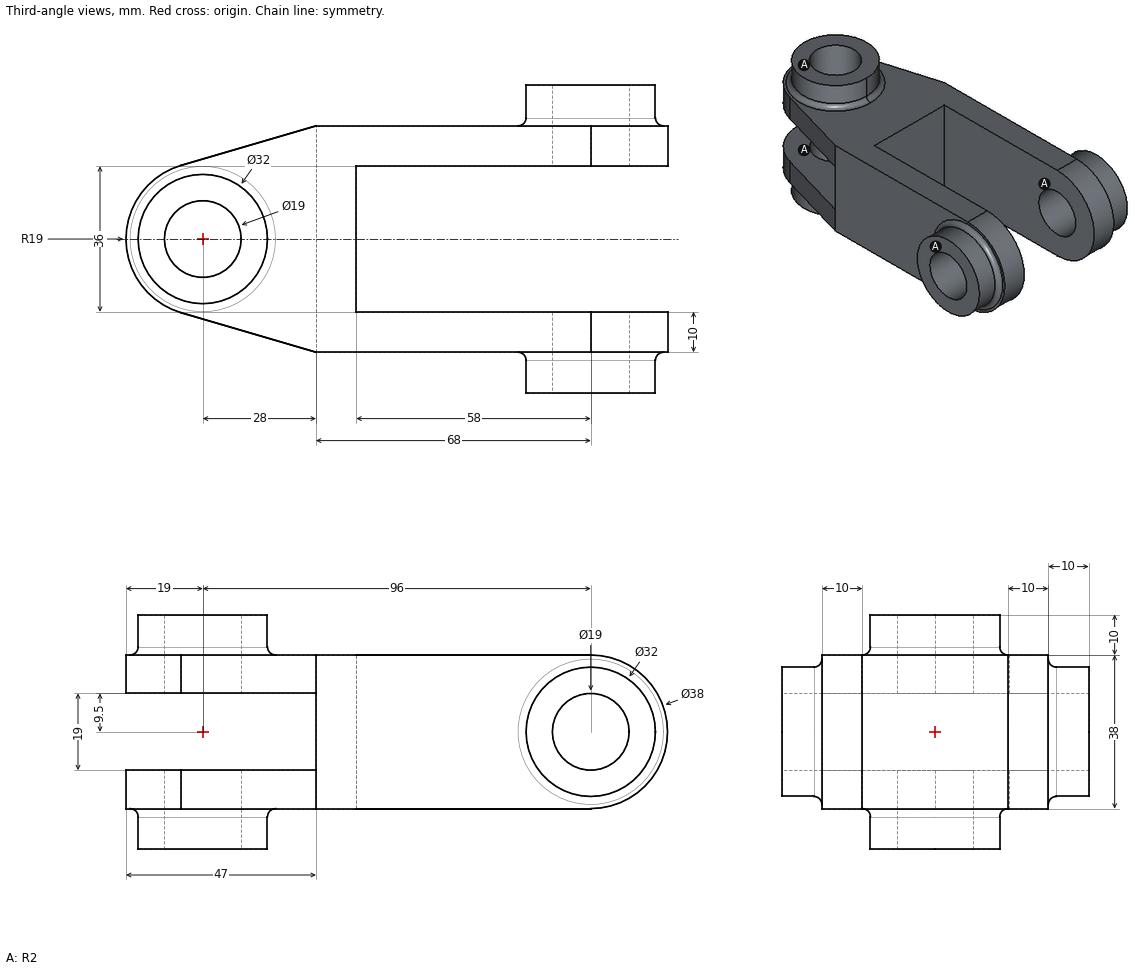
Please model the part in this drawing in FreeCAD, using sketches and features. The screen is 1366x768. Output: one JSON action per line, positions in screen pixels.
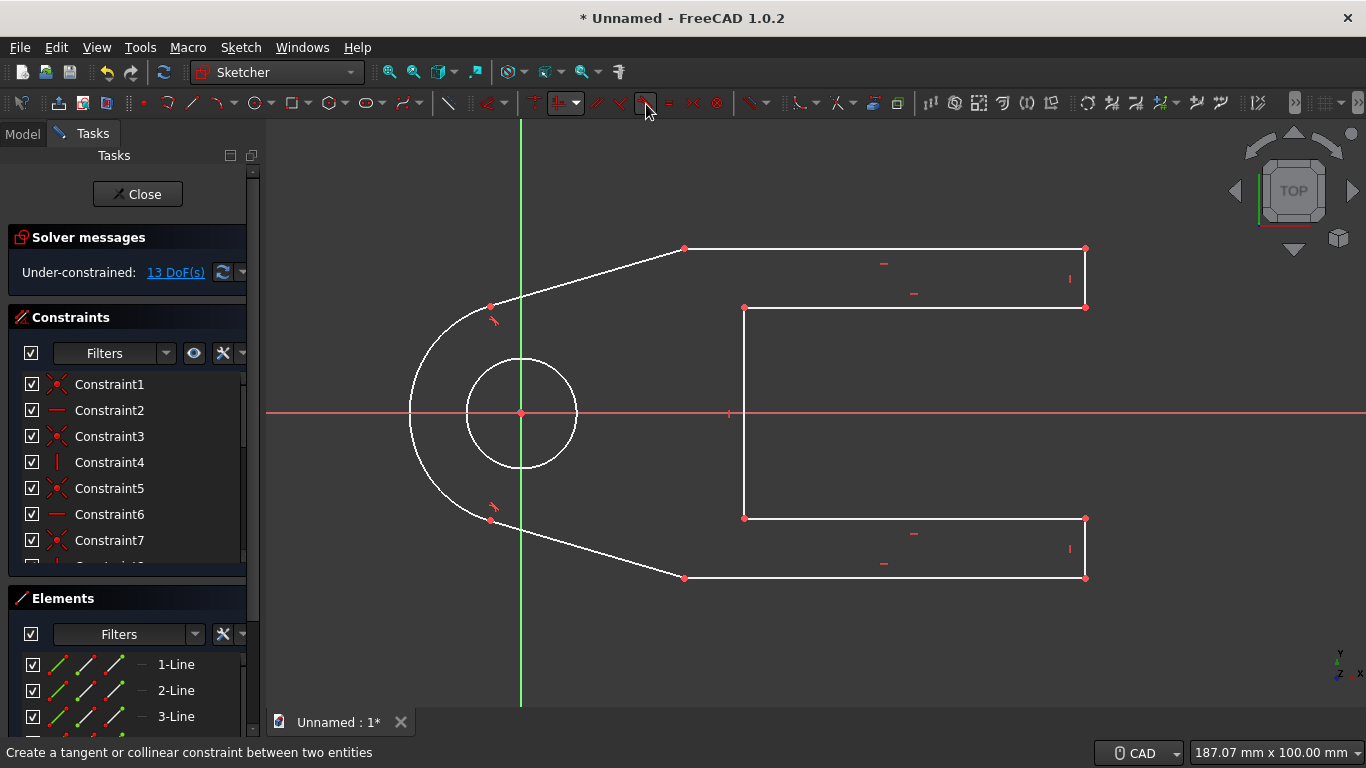
{"action": "left_click_drag", "start_coordinate": [511, 403], "coordinate": [532, 423]}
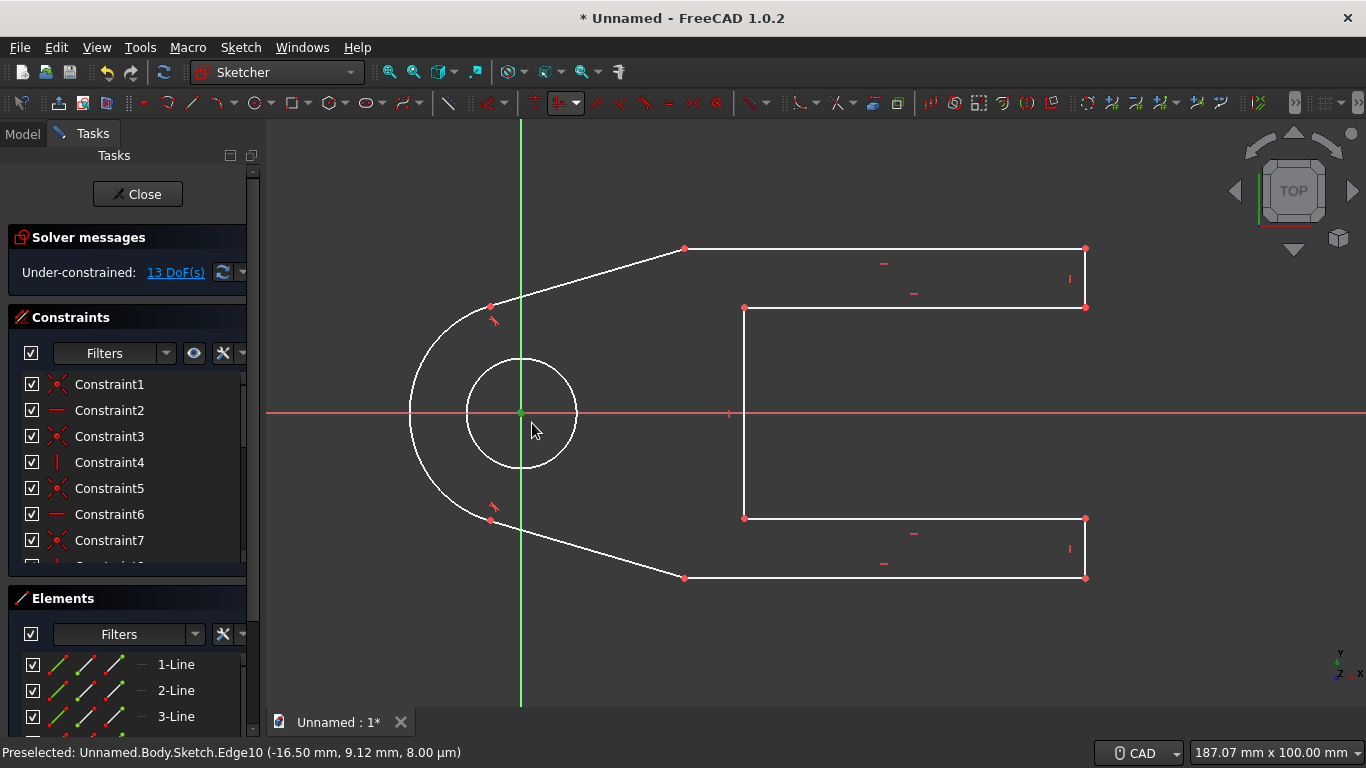
{"action": "key", "text": "c"}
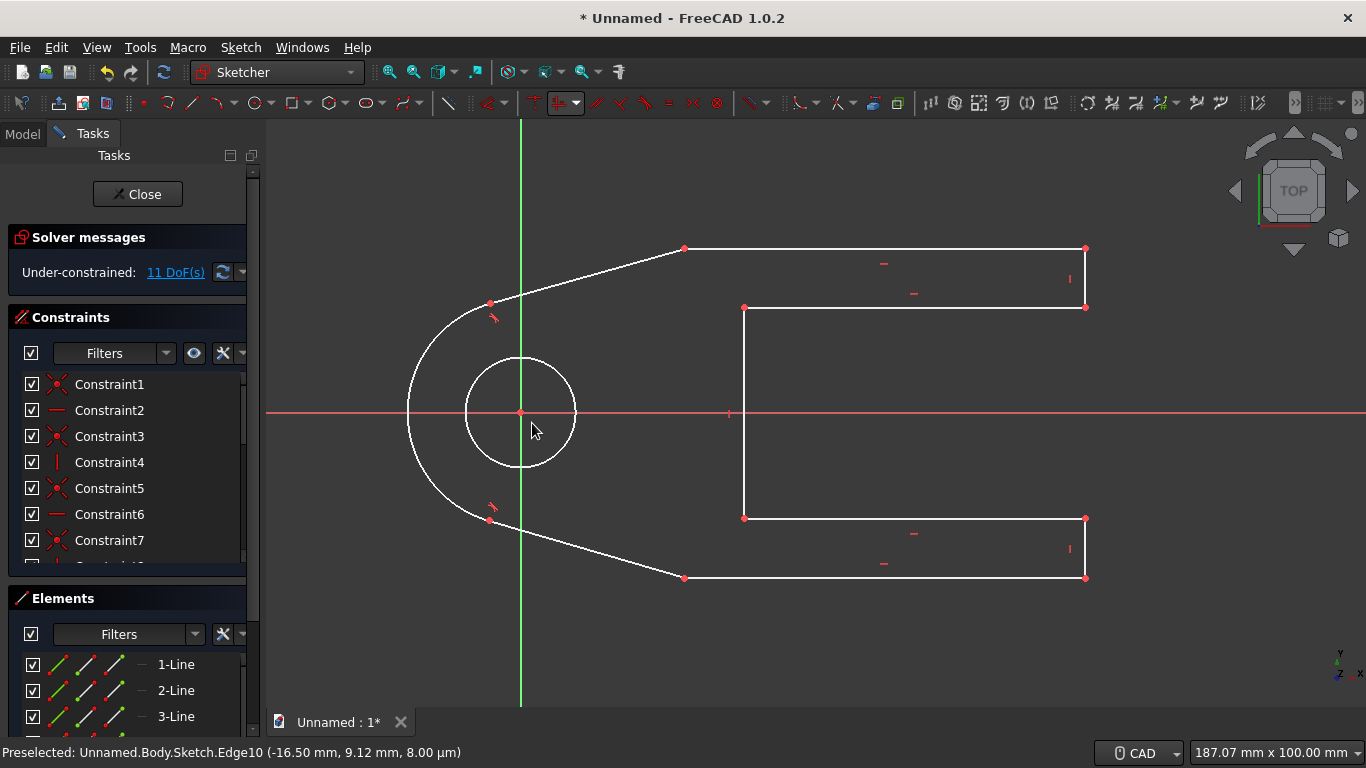
{"action": "left_click", "coordinate": [1085, 519]}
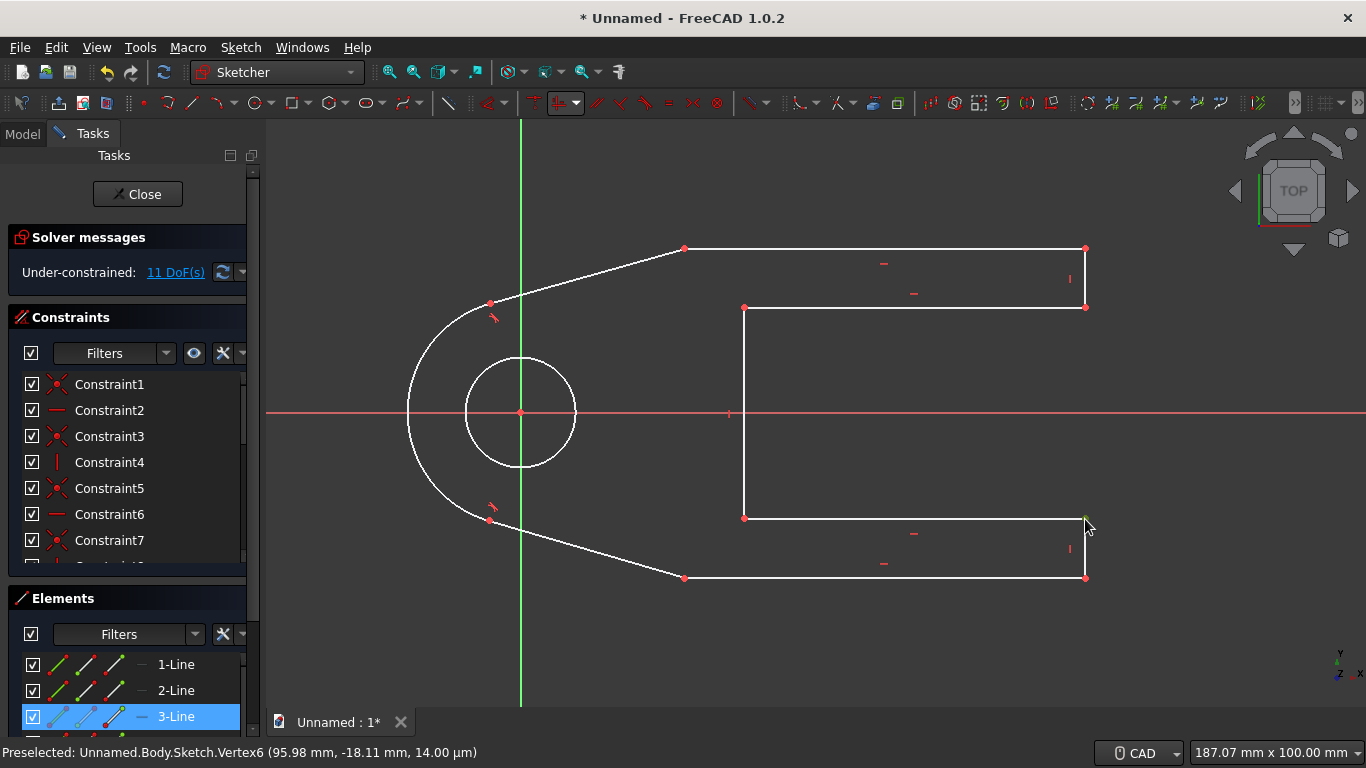
{"action": "left_click", "coordinate": [1085, 308]}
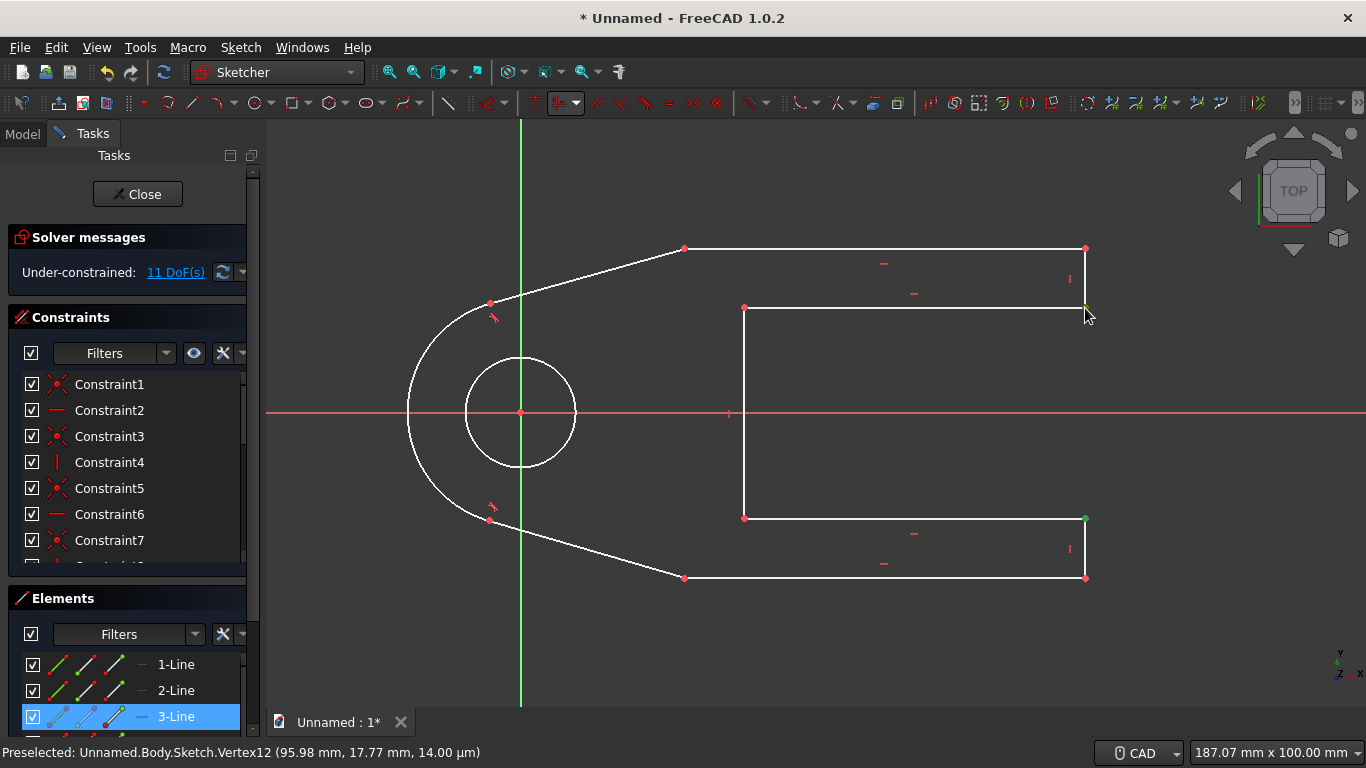
{"action": "left_click", "coordinate": [359, 413]}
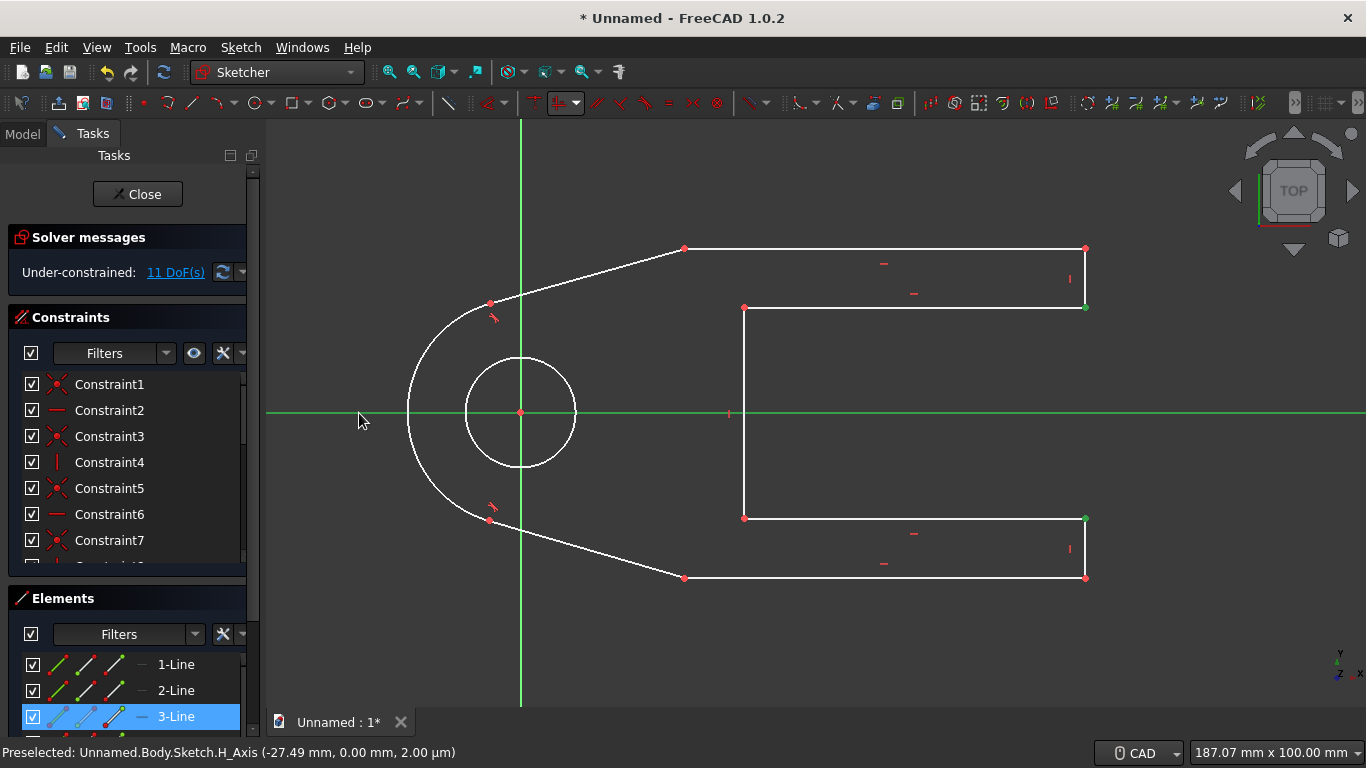
{"action": "key", "text": "s"}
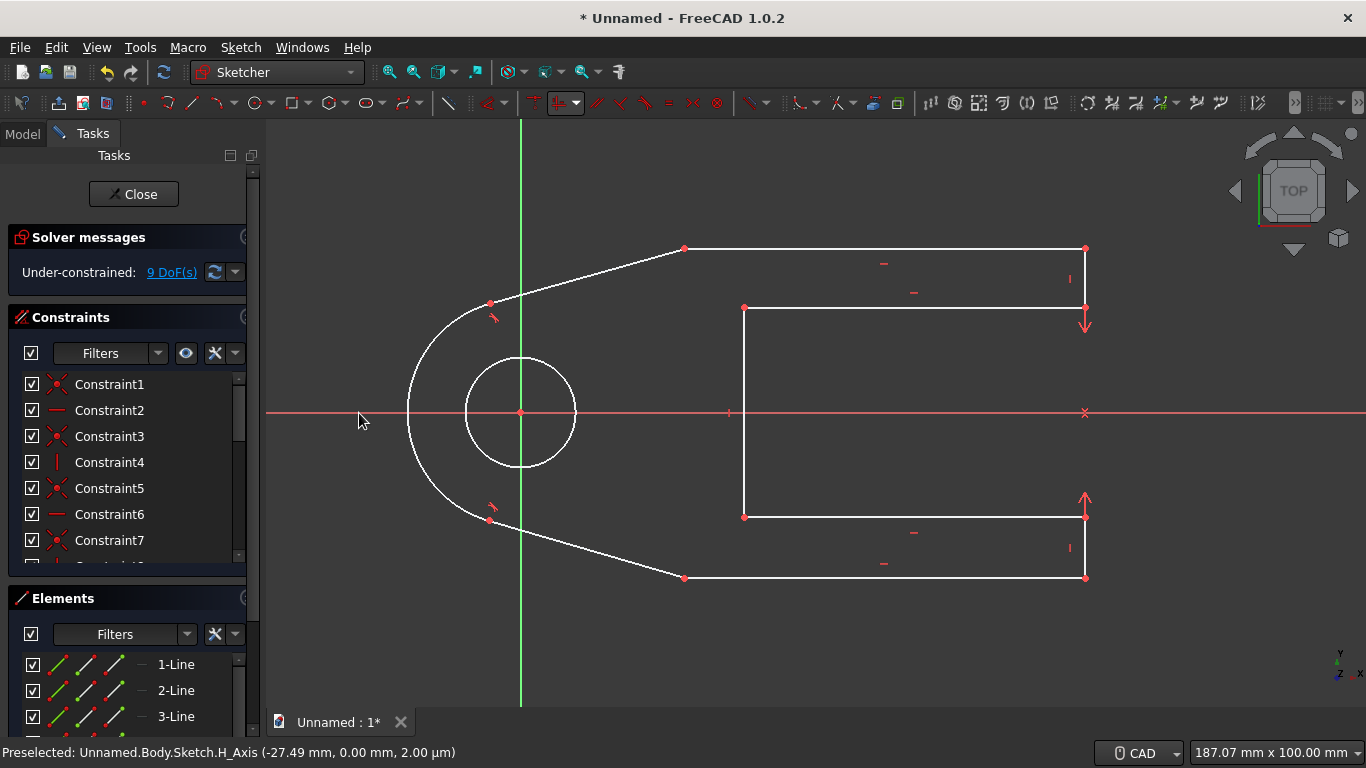
{"action": "left_click", "coordinate": [685, 578]}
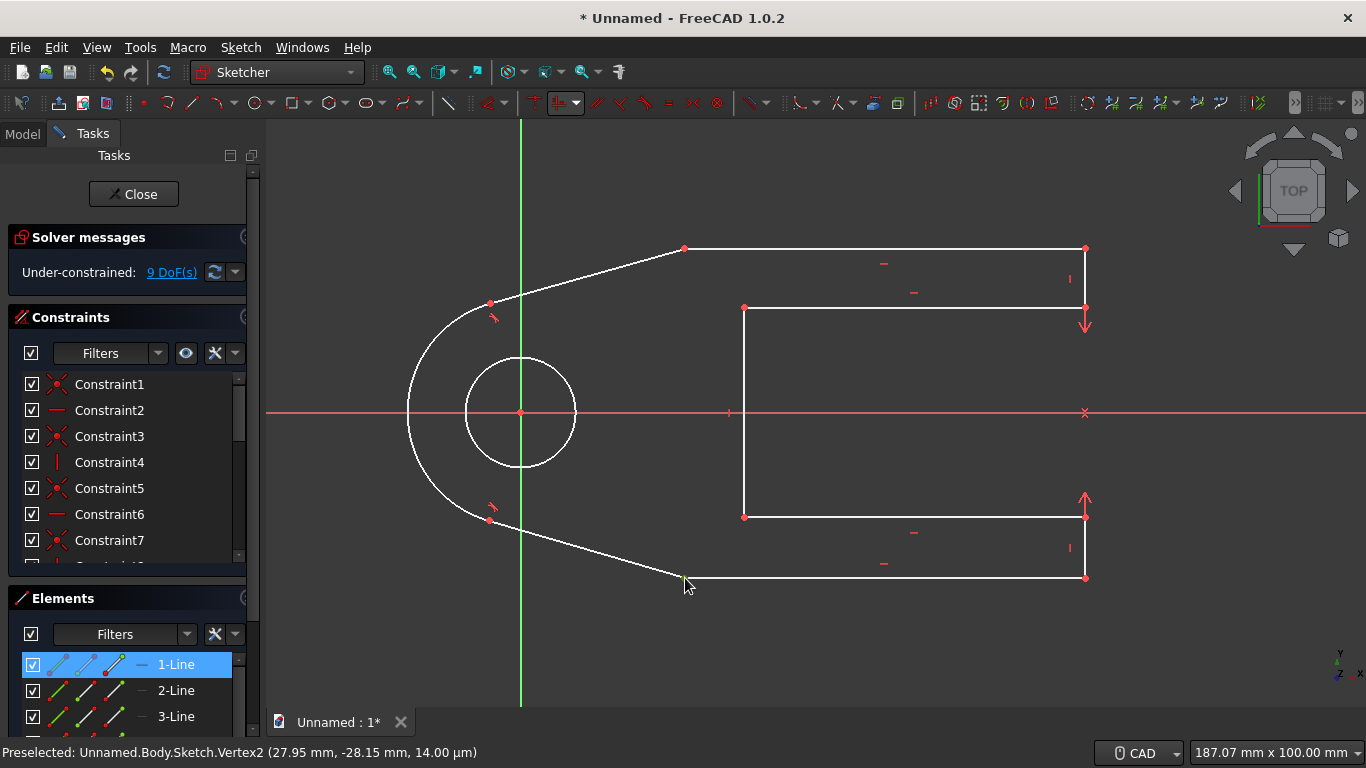
{"action": "left_click", "coordinate": [685, 249]}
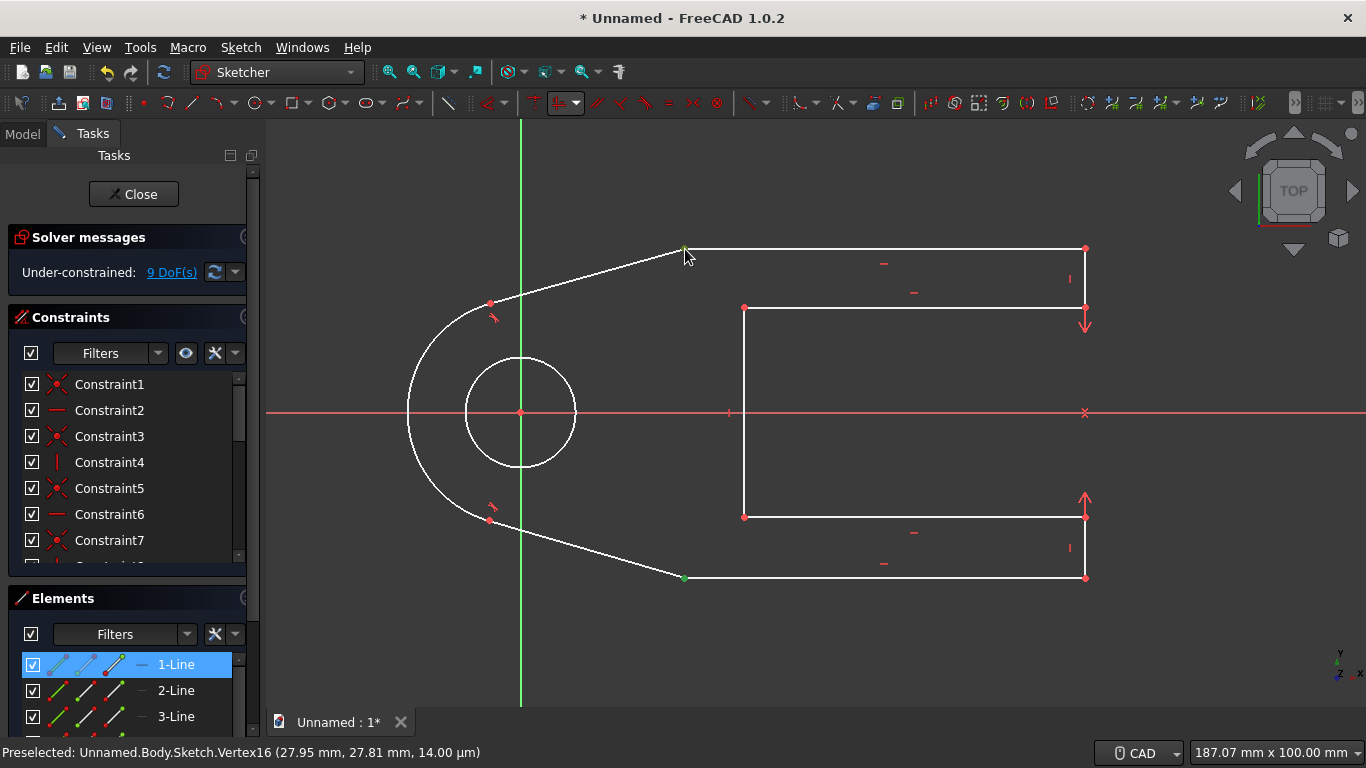
{"action": "left_click", "coordinate": [359, 413]}